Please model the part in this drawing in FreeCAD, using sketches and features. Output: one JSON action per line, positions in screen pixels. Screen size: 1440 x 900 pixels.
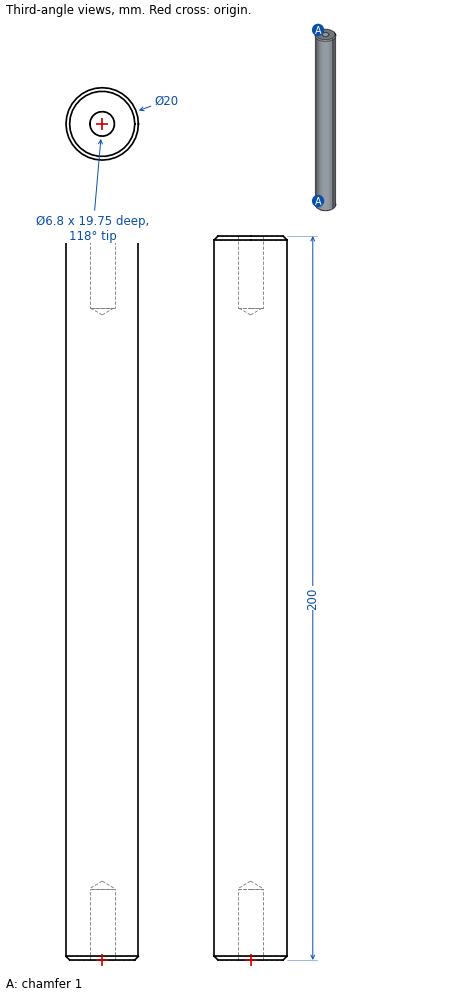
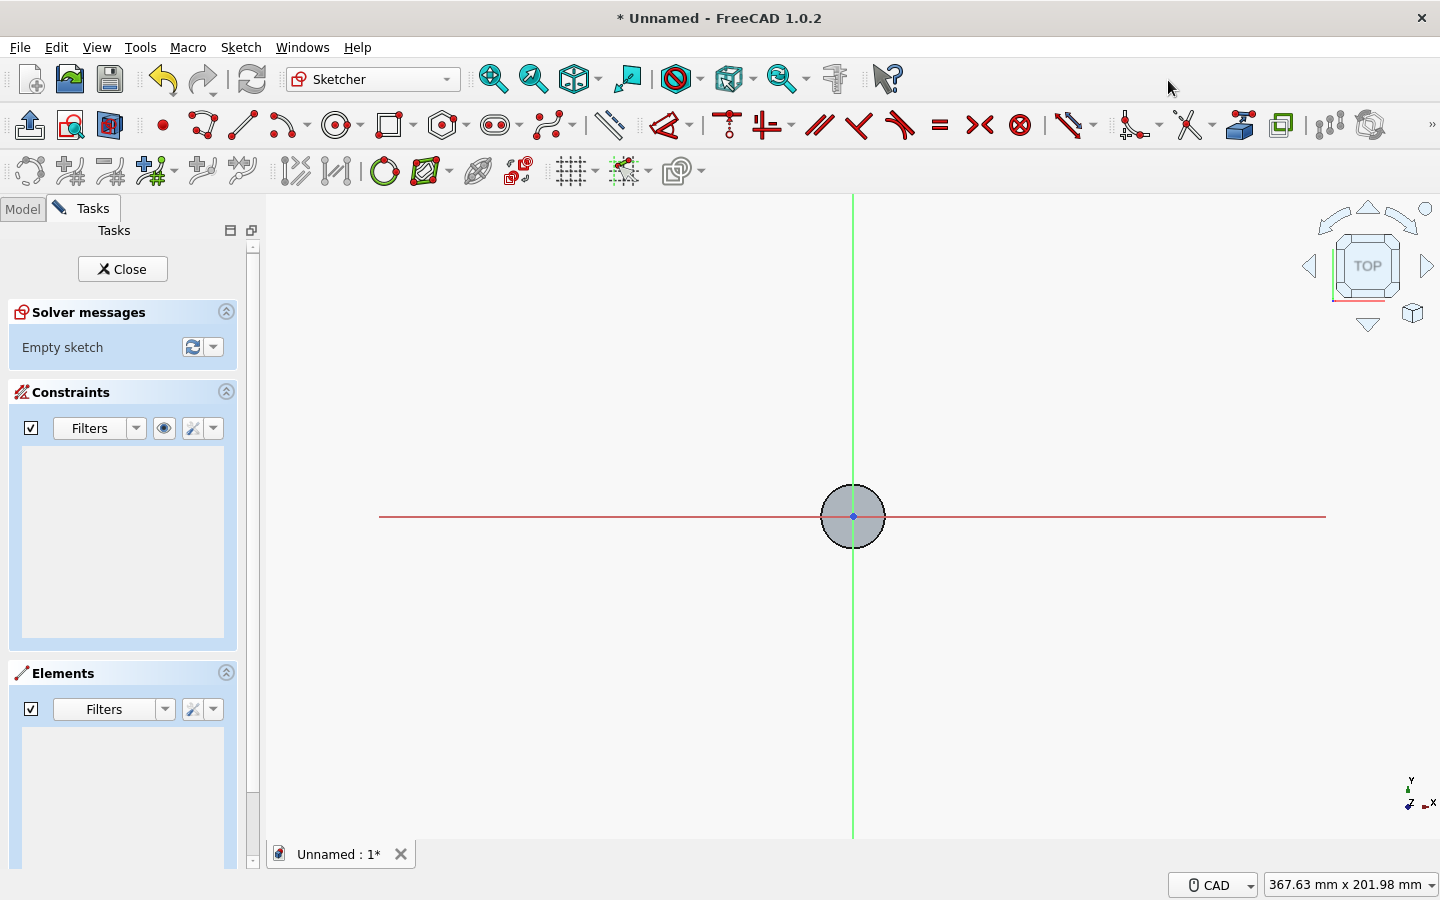
{"action": "scroll", "coordinate": [857, 517], "scroll_direction": "up", "scroll_amount": 15}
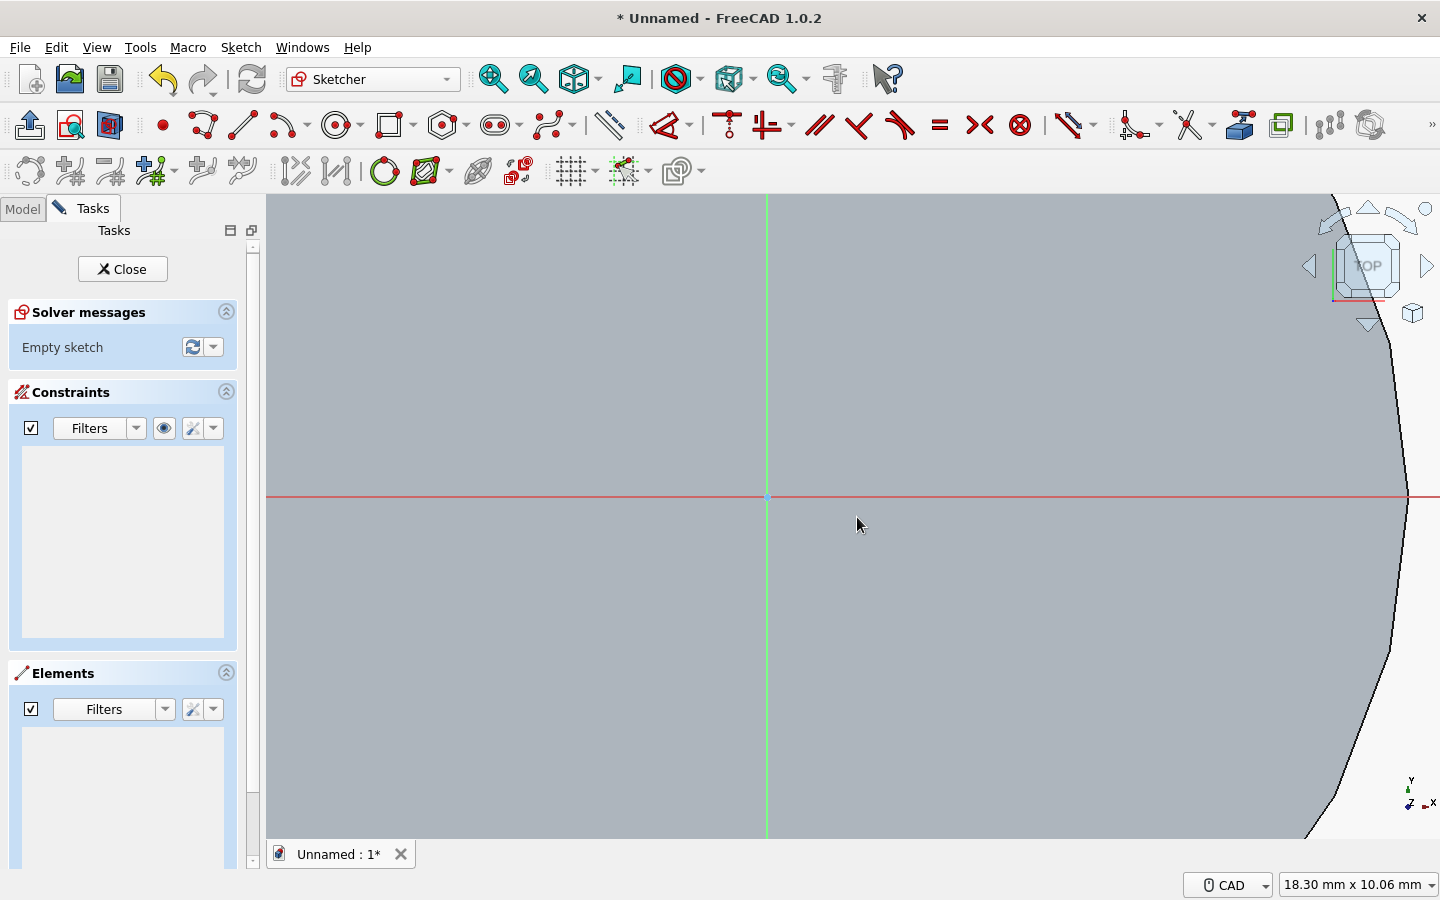
{"action": "key", "text": "g c"}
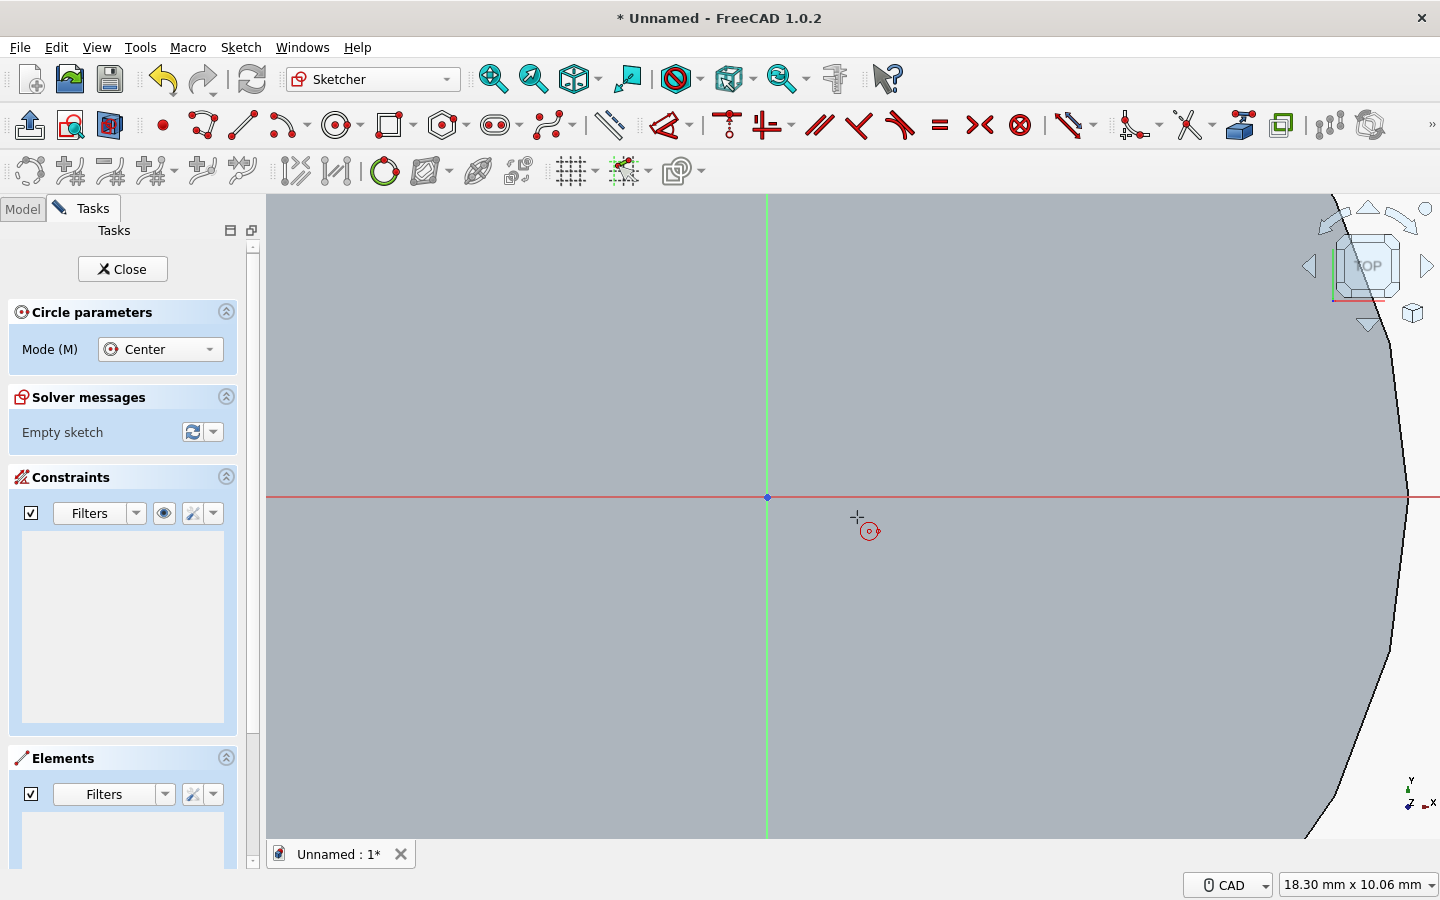
{"action": "left_click", "coordinate": [767, 497]}
{"action": "mouse_move", "coordinate": [921, 343]}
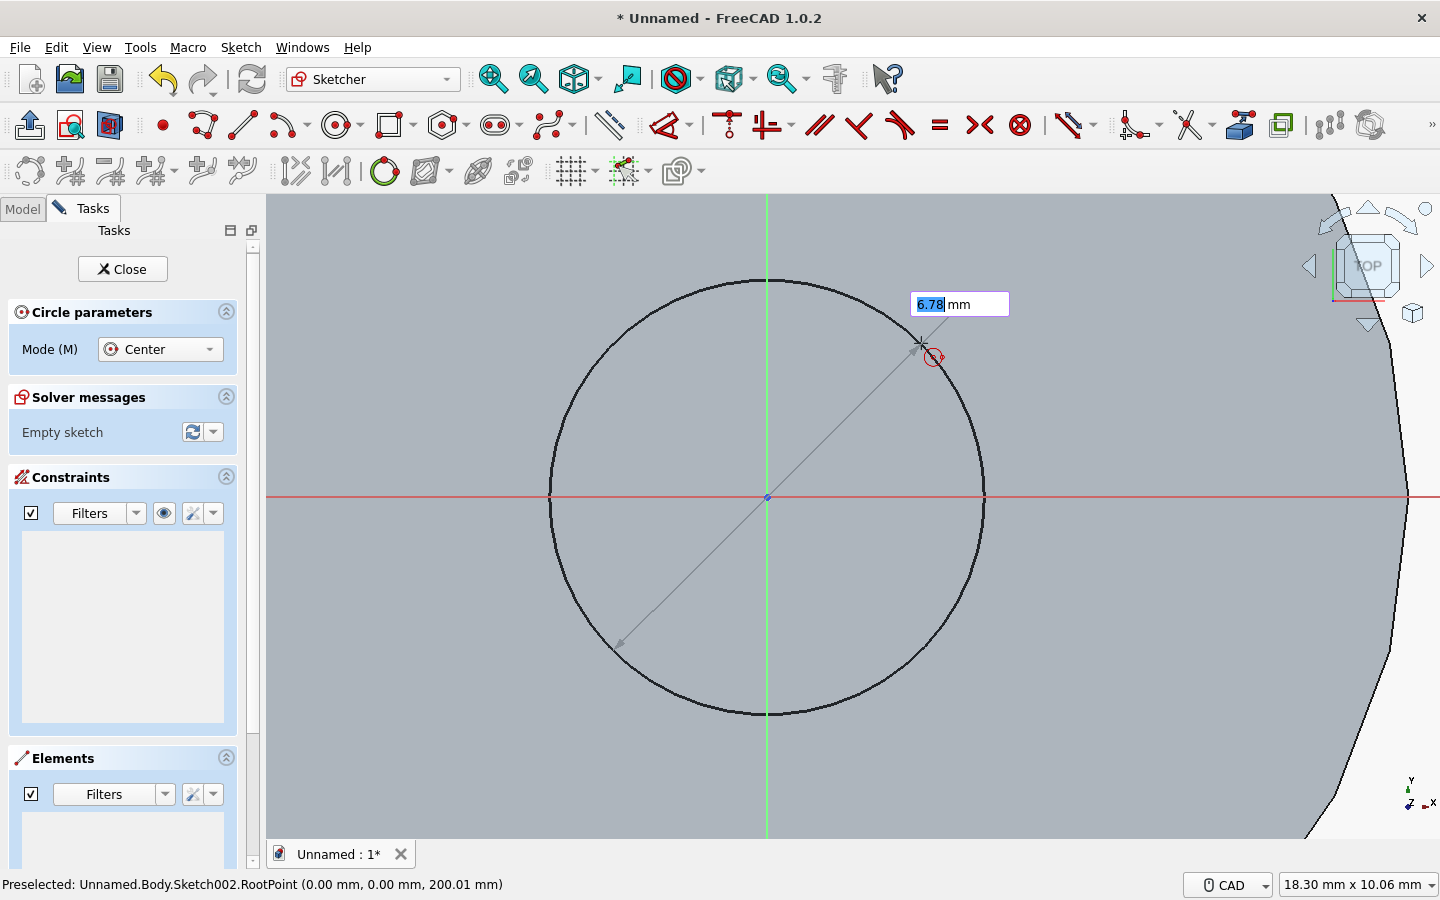
{"action": "type", "text": "6.8"}
{"action": "key", "text": "Return"}
{"action": "key", "text": "Escape"}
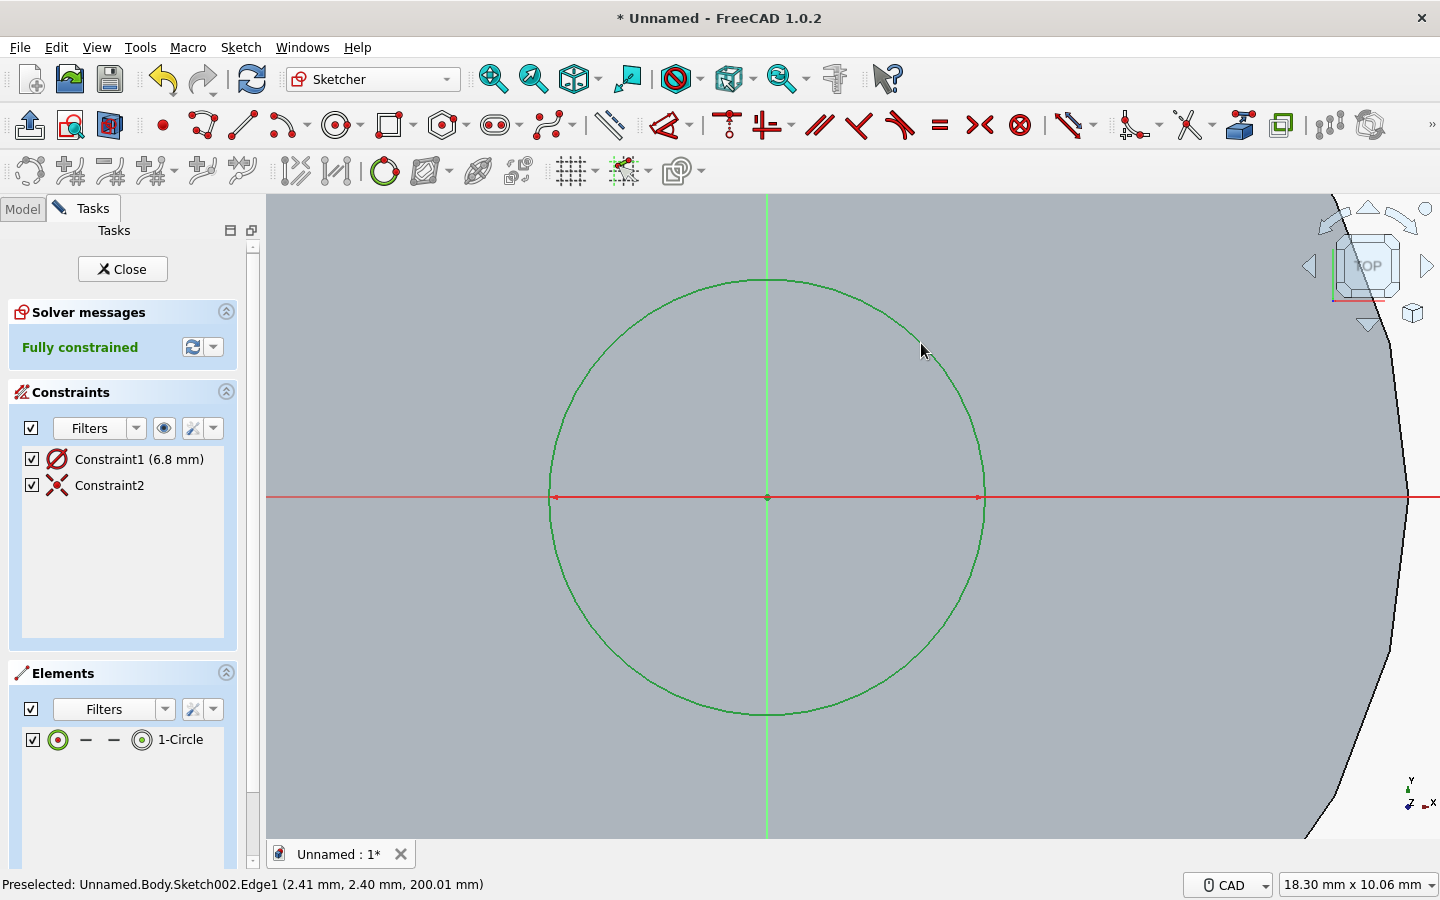
{"action": "left_click", "coordinate": [123, 269]}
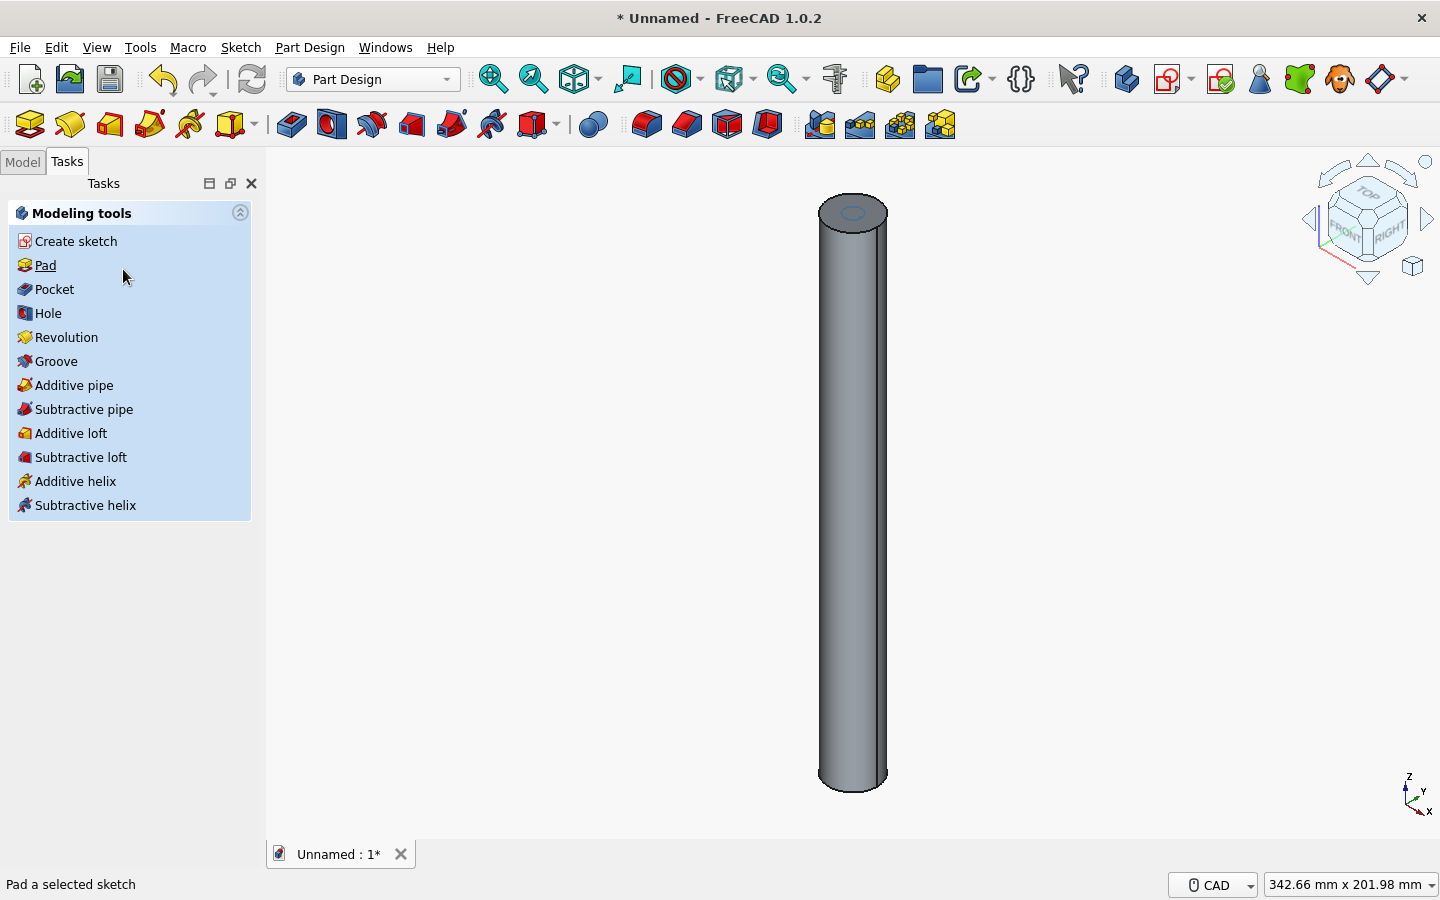
{"action": "left_click", "coordinate": [332, 124]}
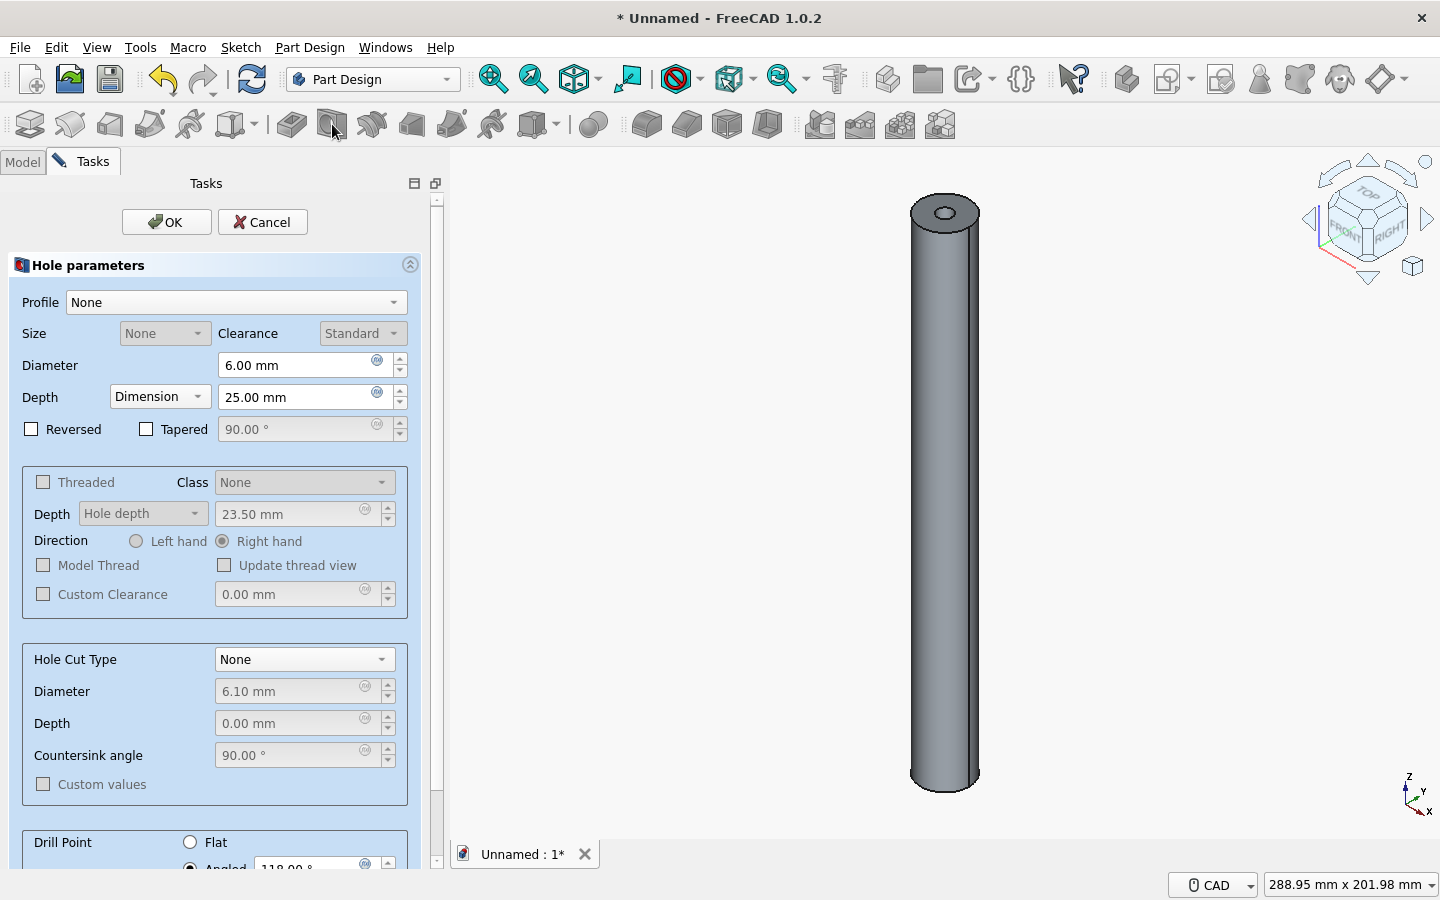
{"action": "triple_click", "coordinate": [305, 365]}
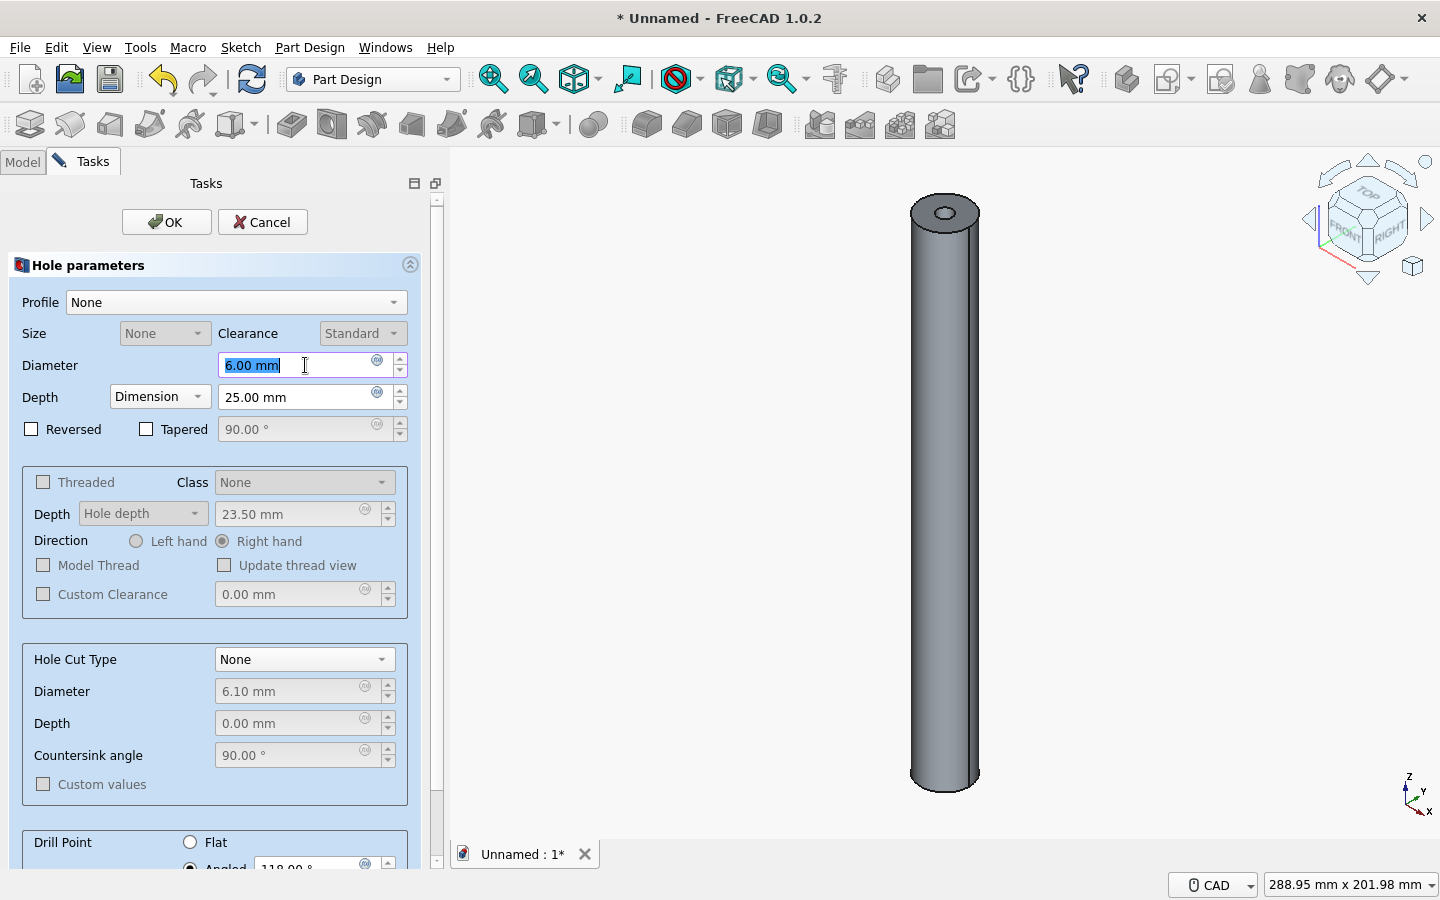
{"action": "type", "text": "6.8"}
{"action": "key", "text": "Tab"}